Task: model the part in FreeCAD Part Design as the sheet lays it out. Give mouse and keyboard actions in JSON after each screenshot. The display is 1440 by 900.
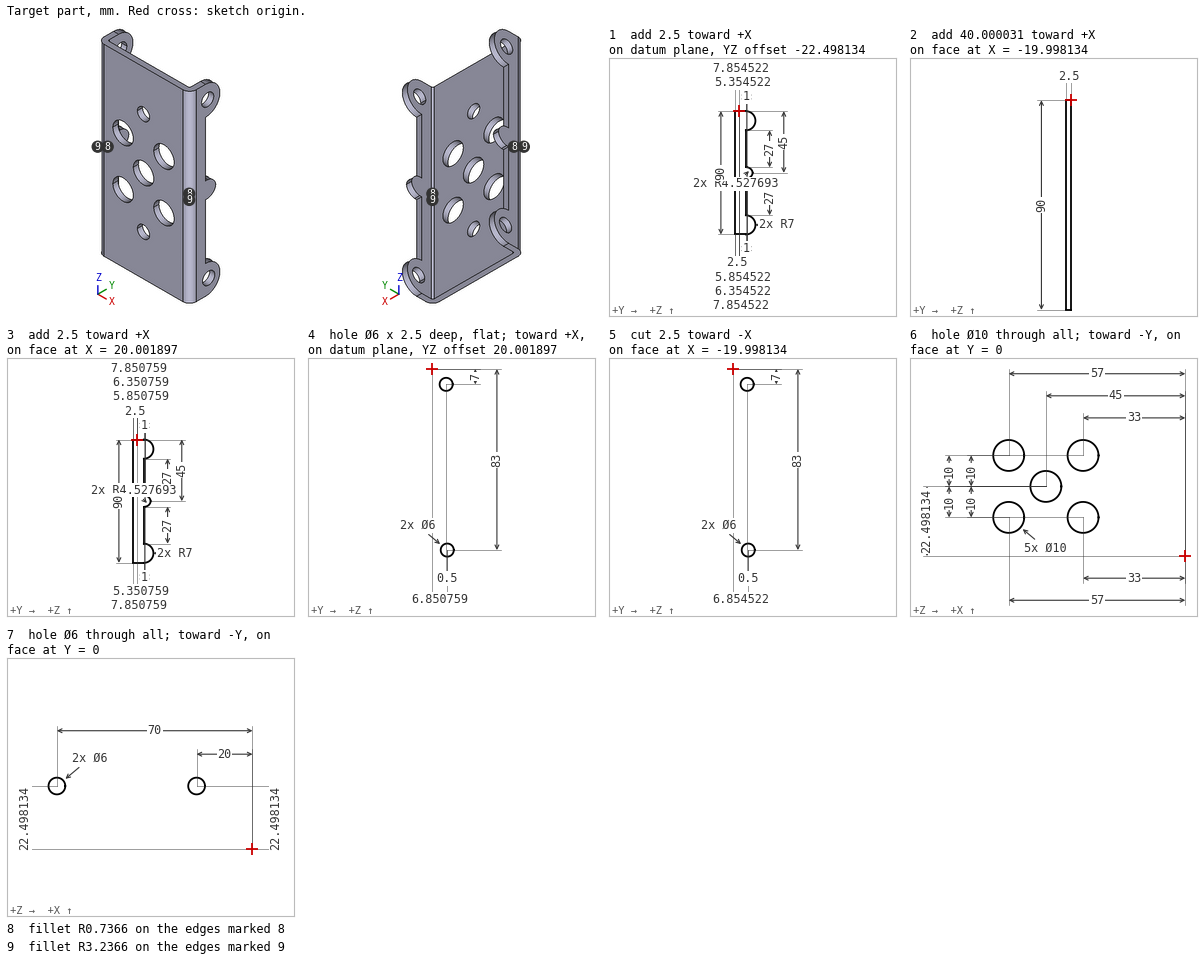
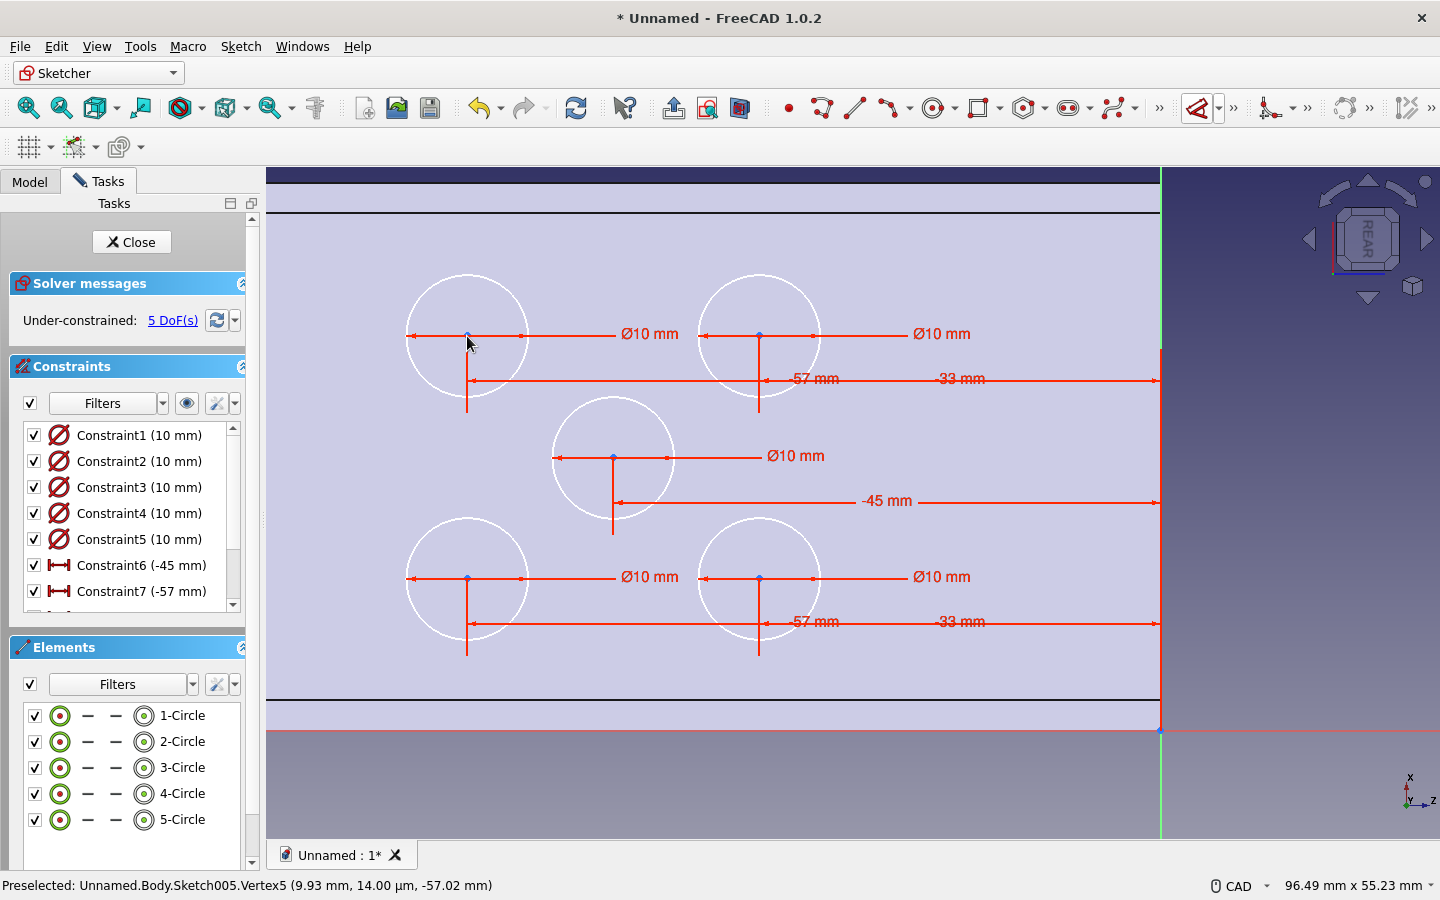
{"action": "left_click", "coordinate": [613, 458]}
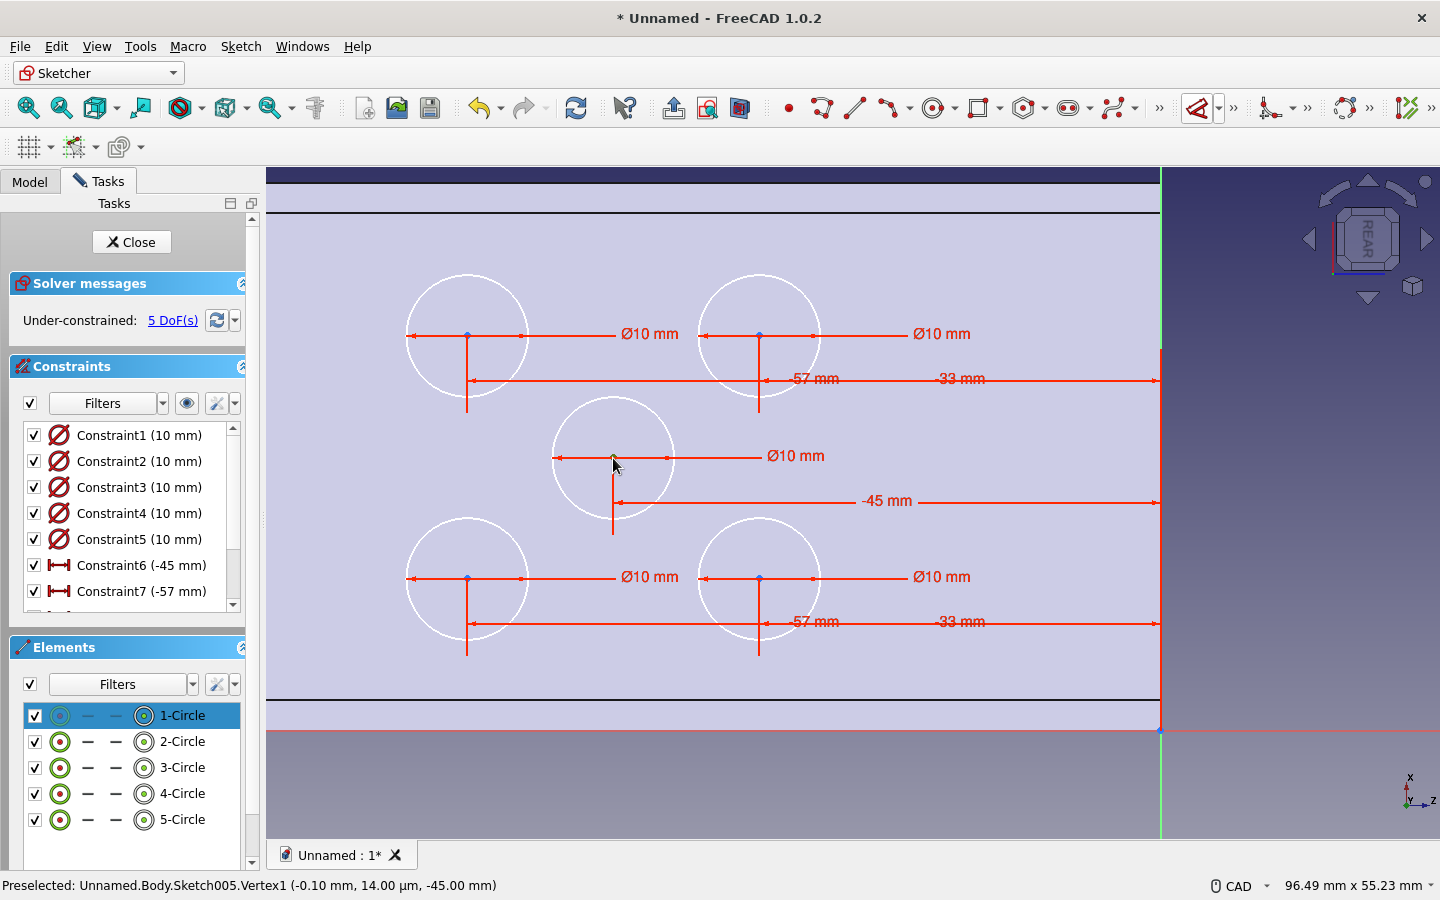
{"action": "left_click", "coordinate": [467, 579]}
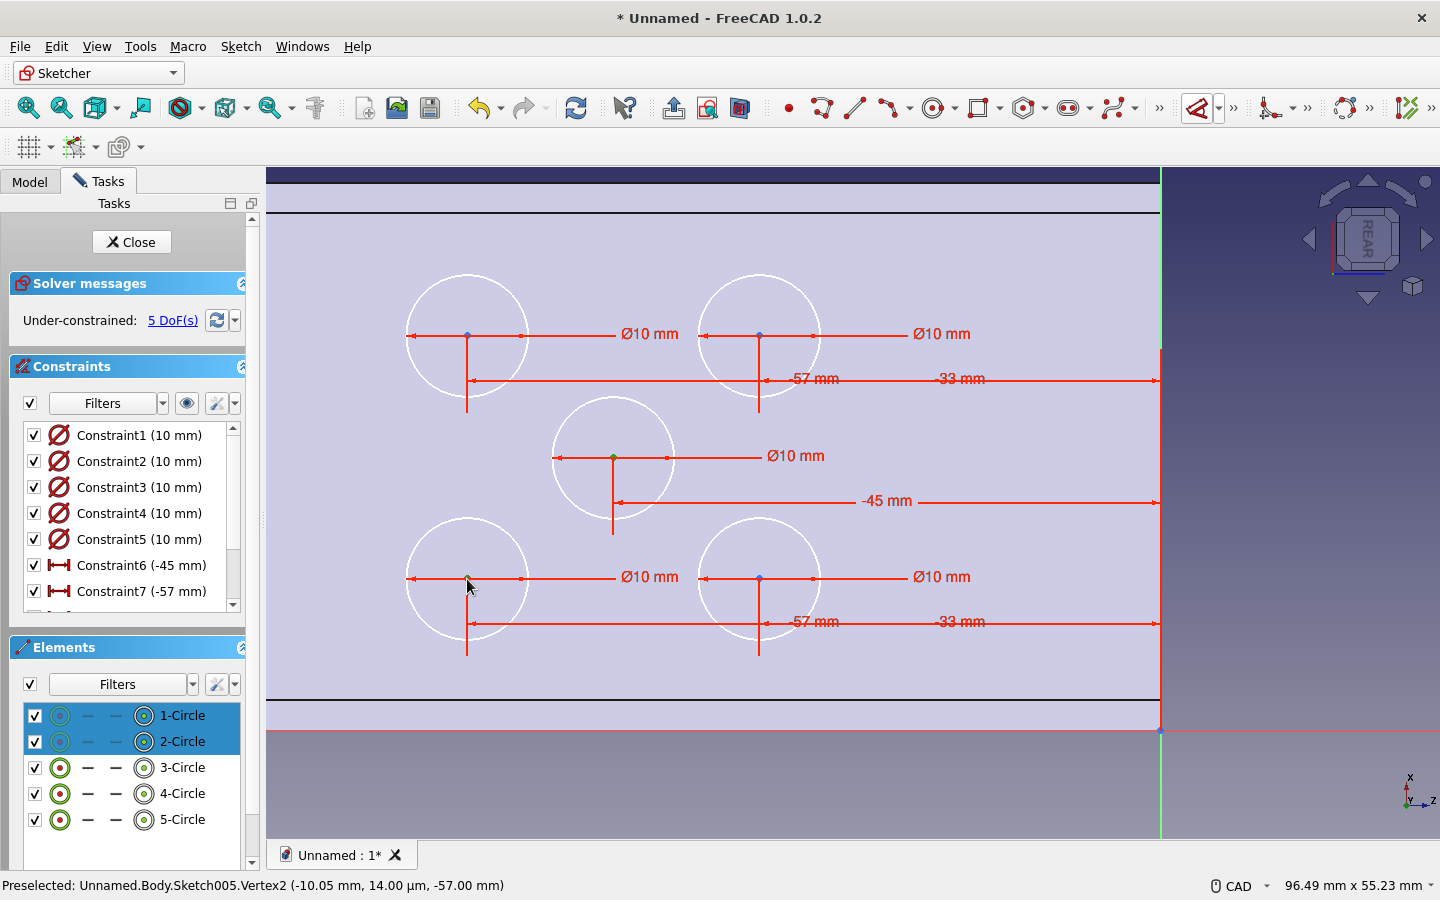
{"action": "left_click", "coordinate": [1218, 108]}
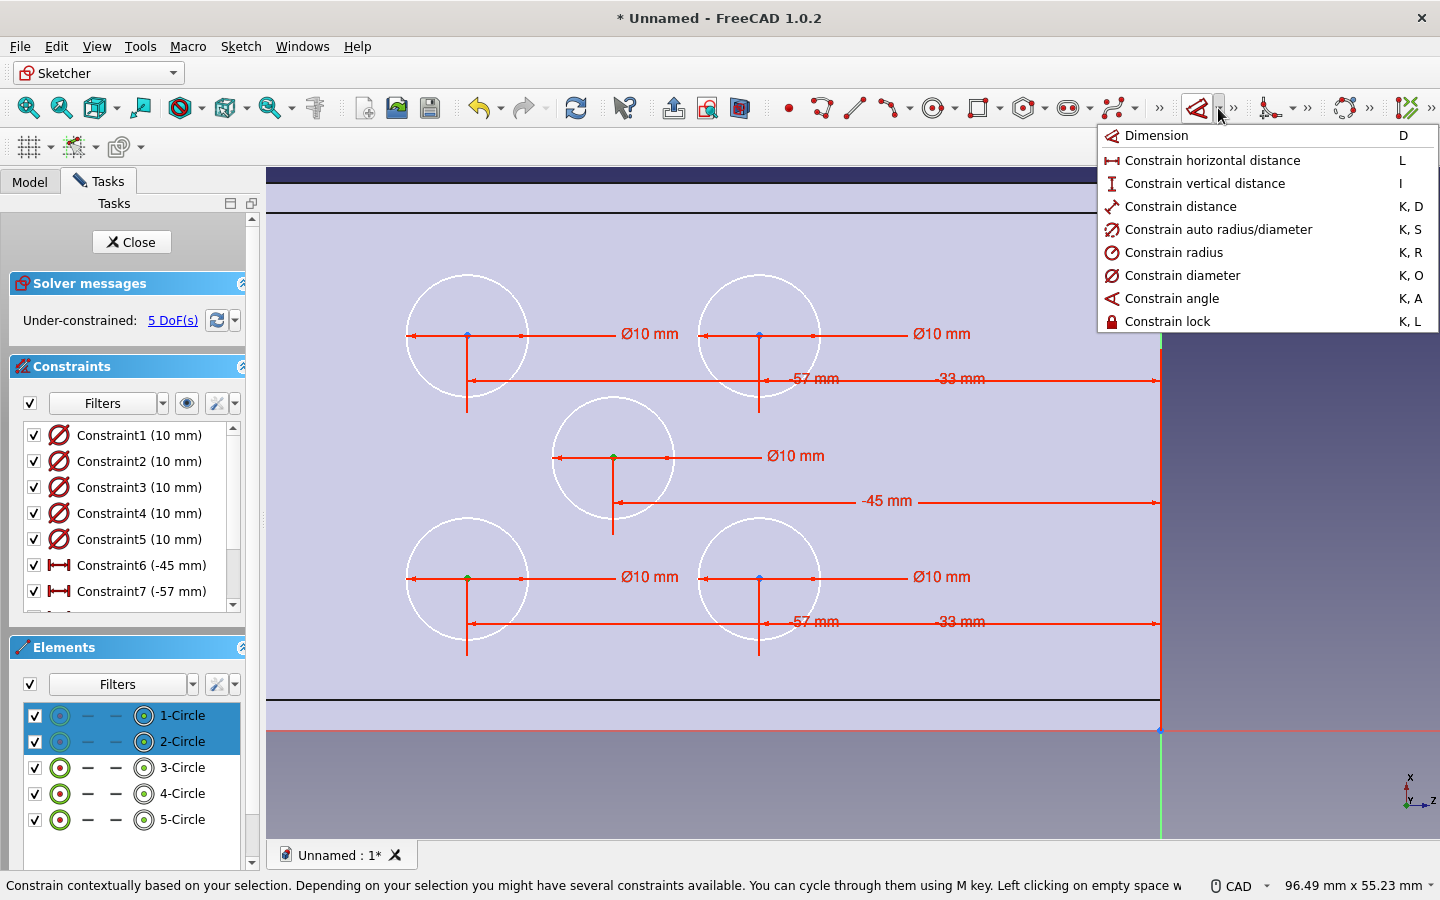
{"action": "left_click", "coordinate": [1268, 184]}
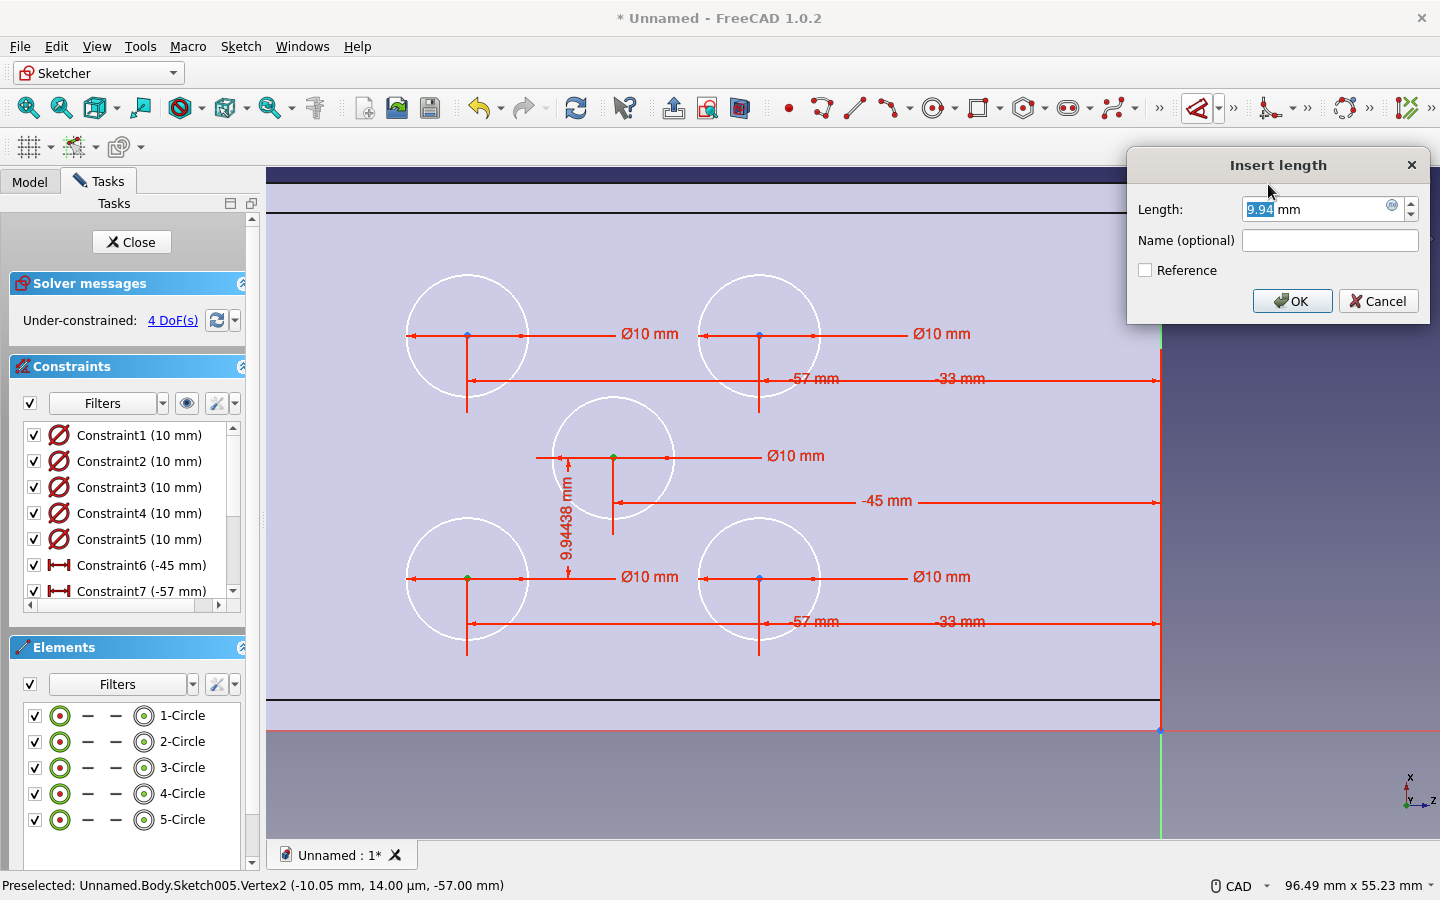
{"action": "type", "text": "10"}
{"action": "key", "text": "Return"}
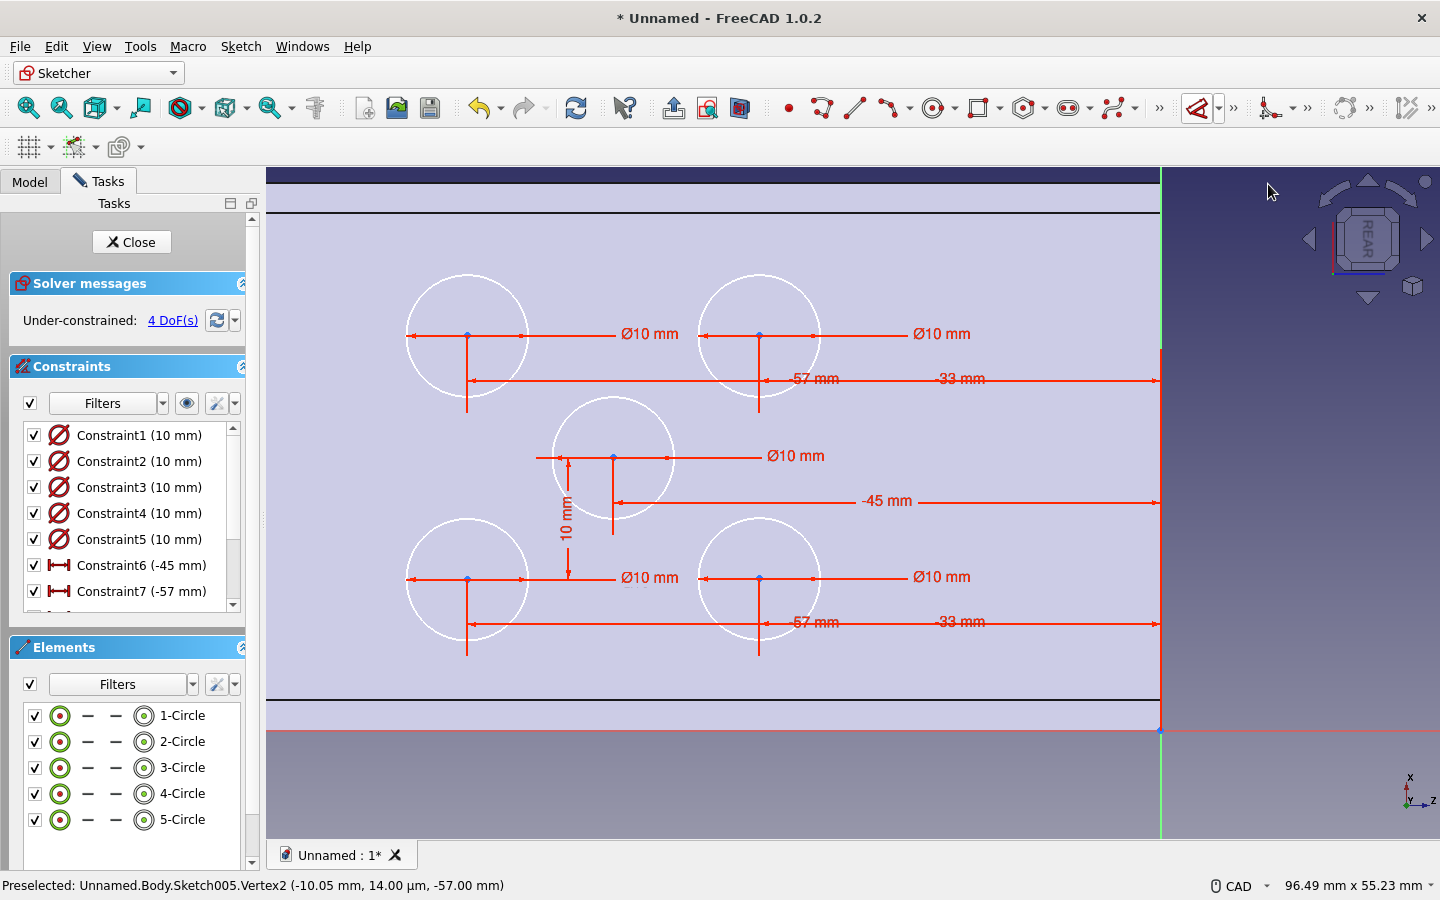
{"action": "left_click", "coordinate": [613, 458]}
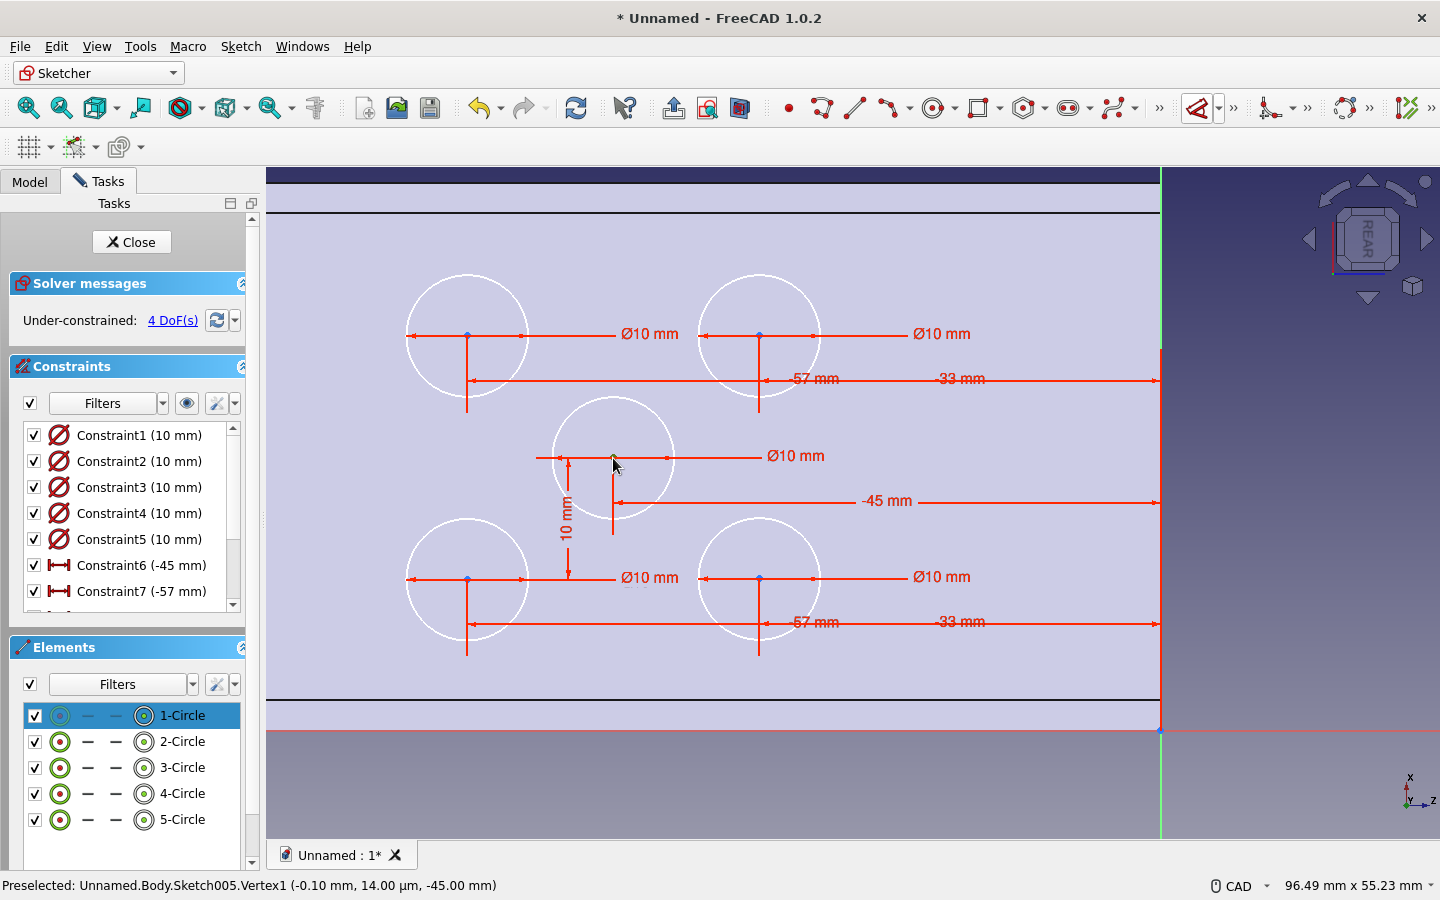
{"action": "left_click", "coordinate": [759, 579]}